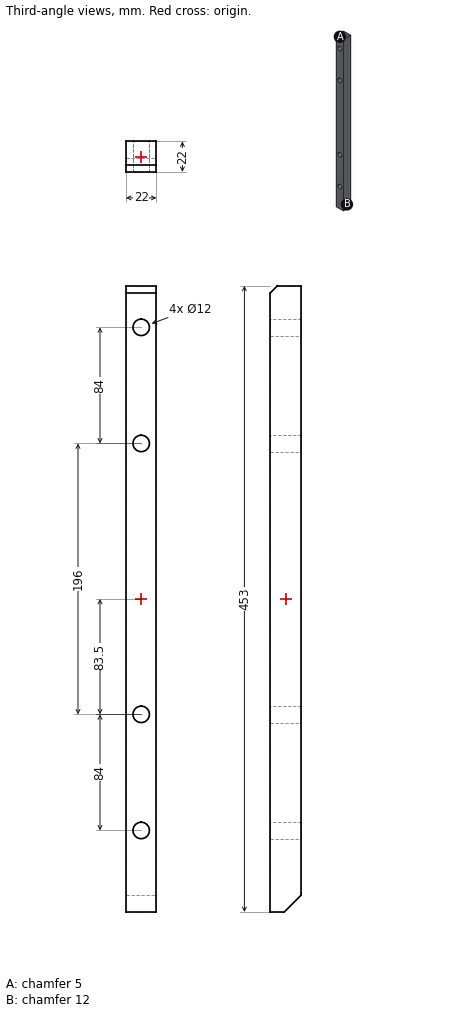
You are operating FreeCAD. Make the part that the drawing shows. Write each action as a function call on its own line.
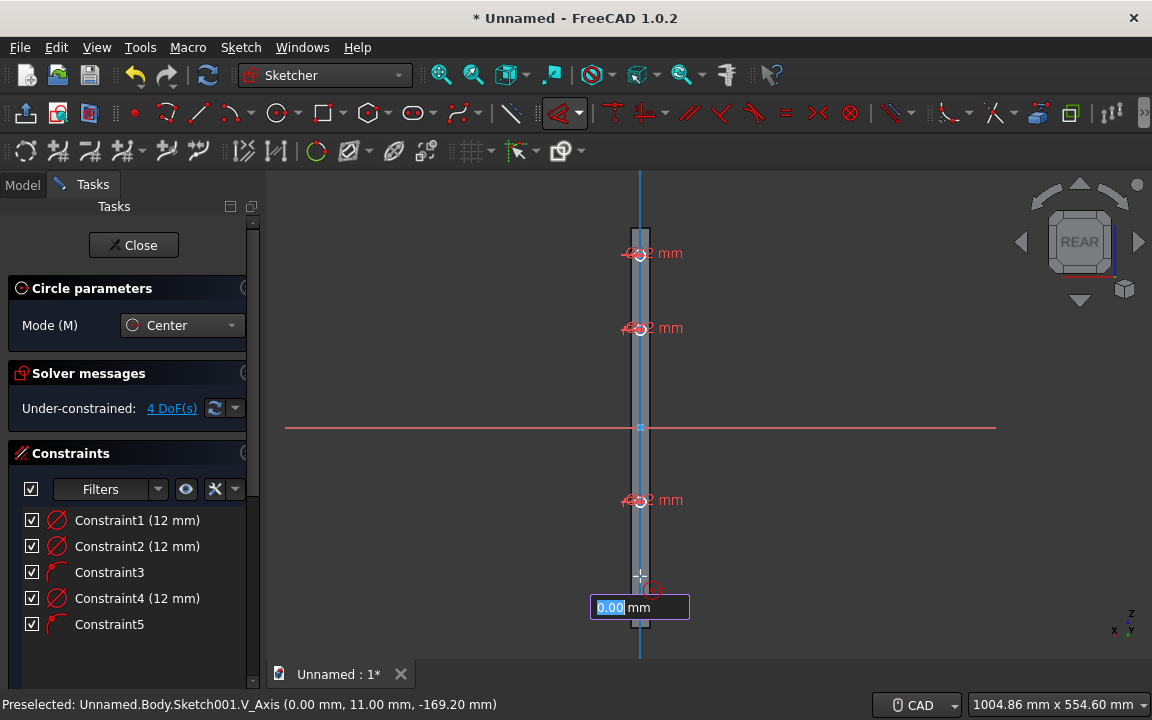
scroll(645, 574, up, 6)
move(646, 571)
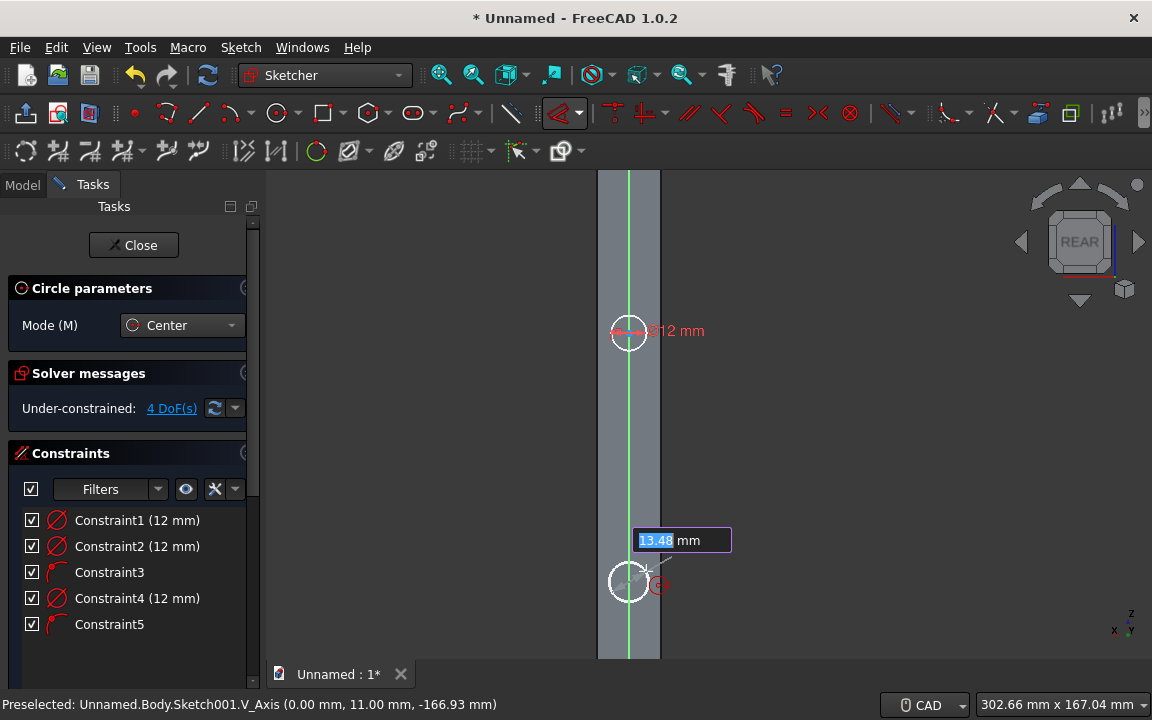
text(12)
key(Return)
key(Escape)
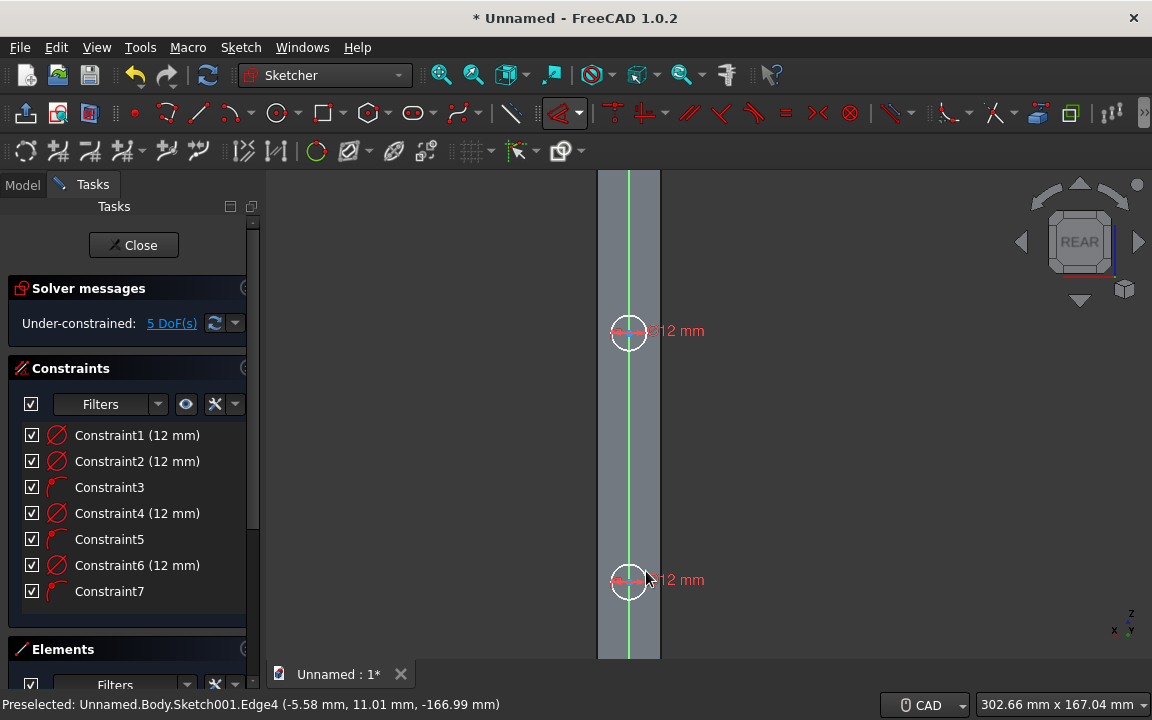
scroll(645, 574, down, 6)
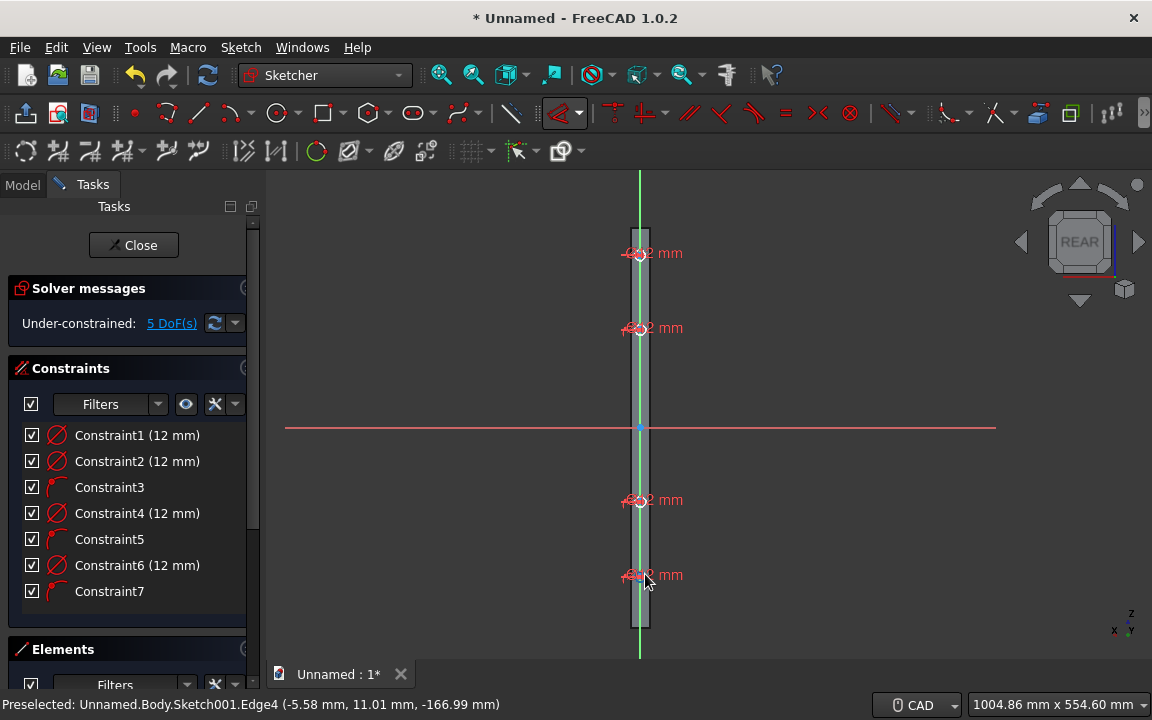
click(640, 255)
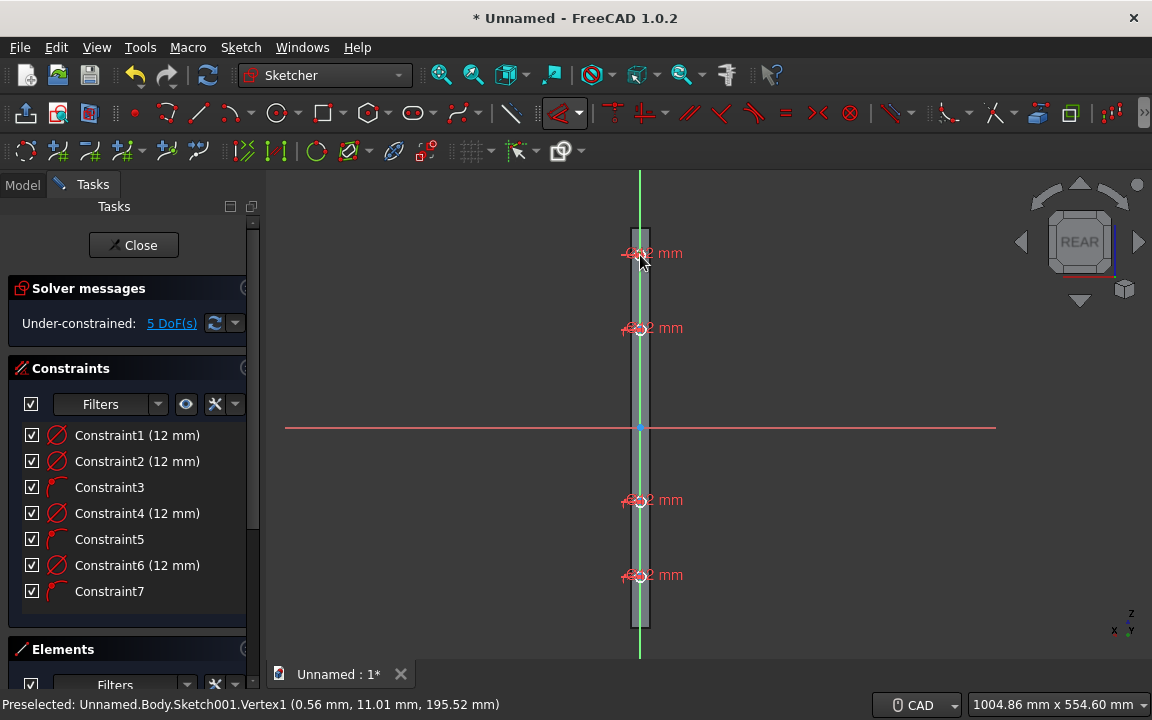
click(640, 538)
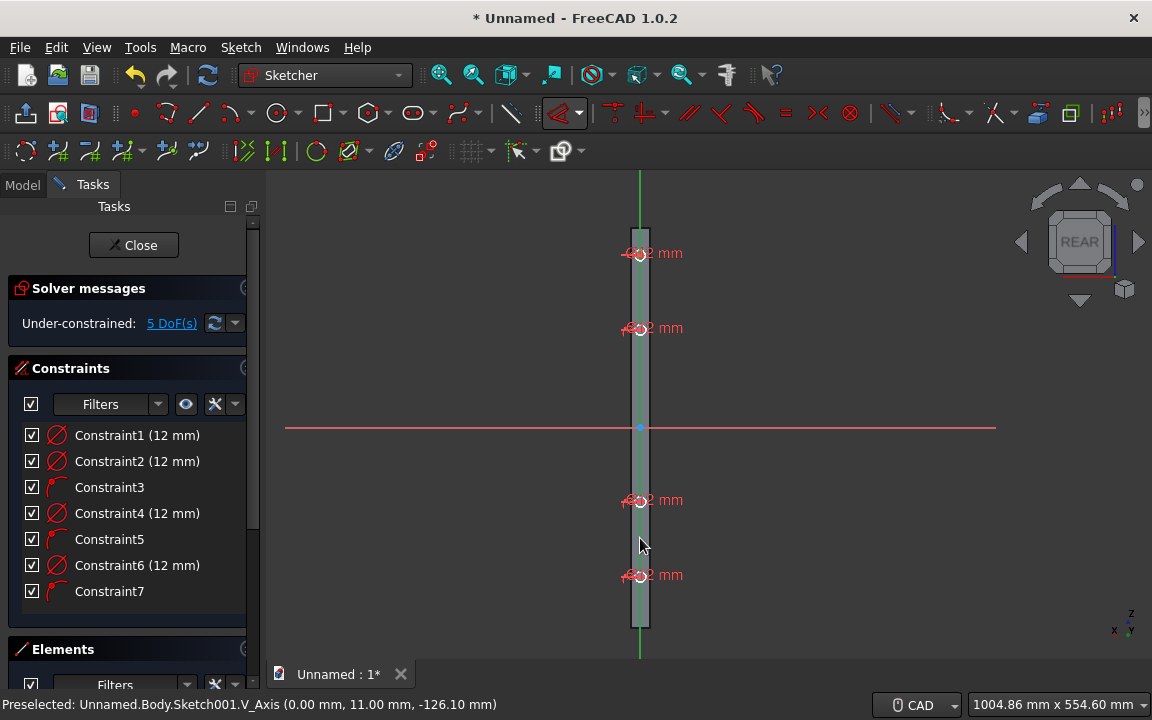
key(c)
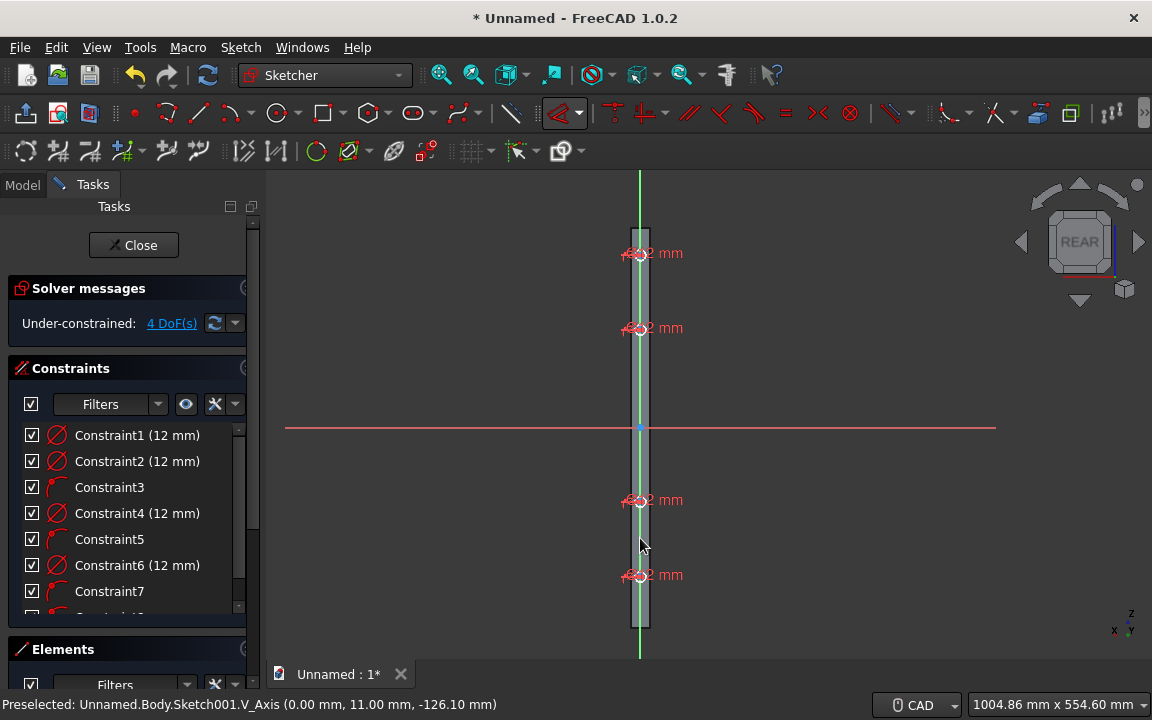
key(d)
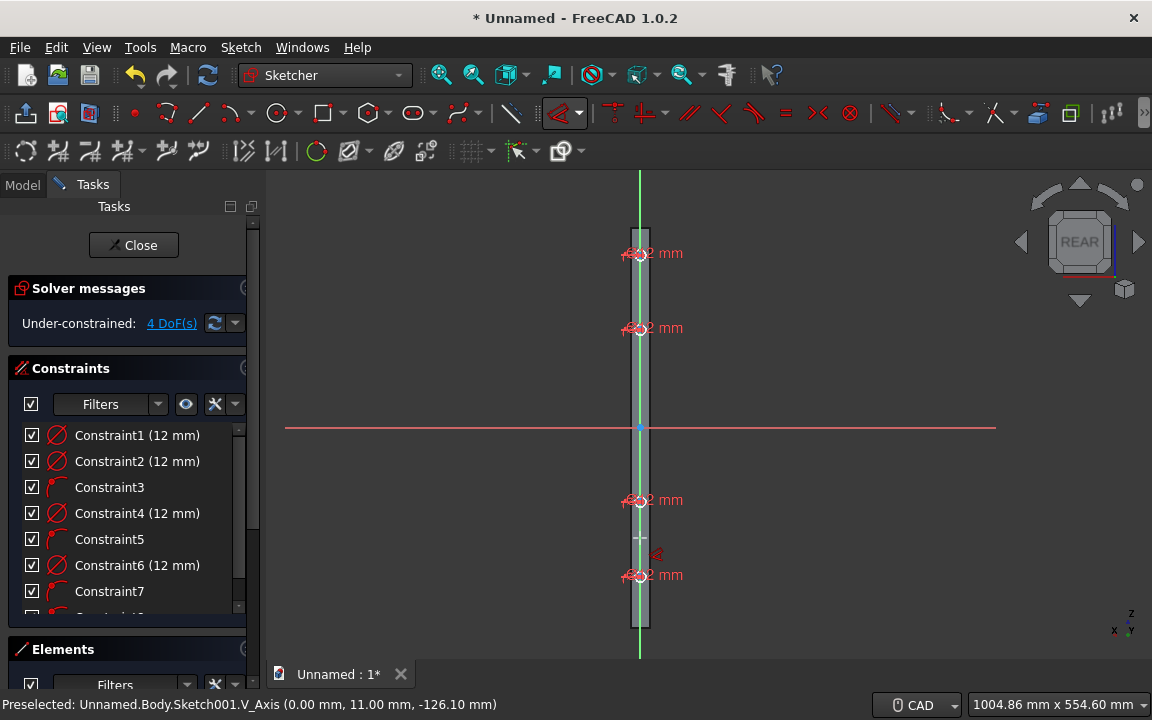
click(640, 255)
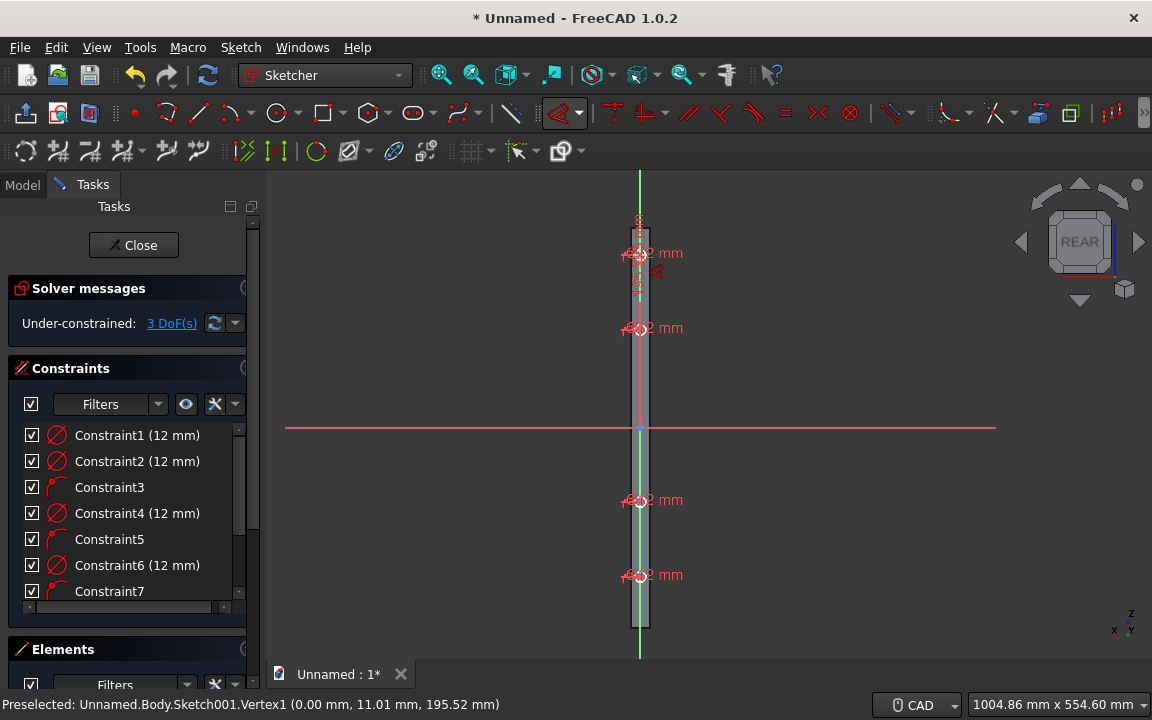
click(640, 330)
click(674, 293)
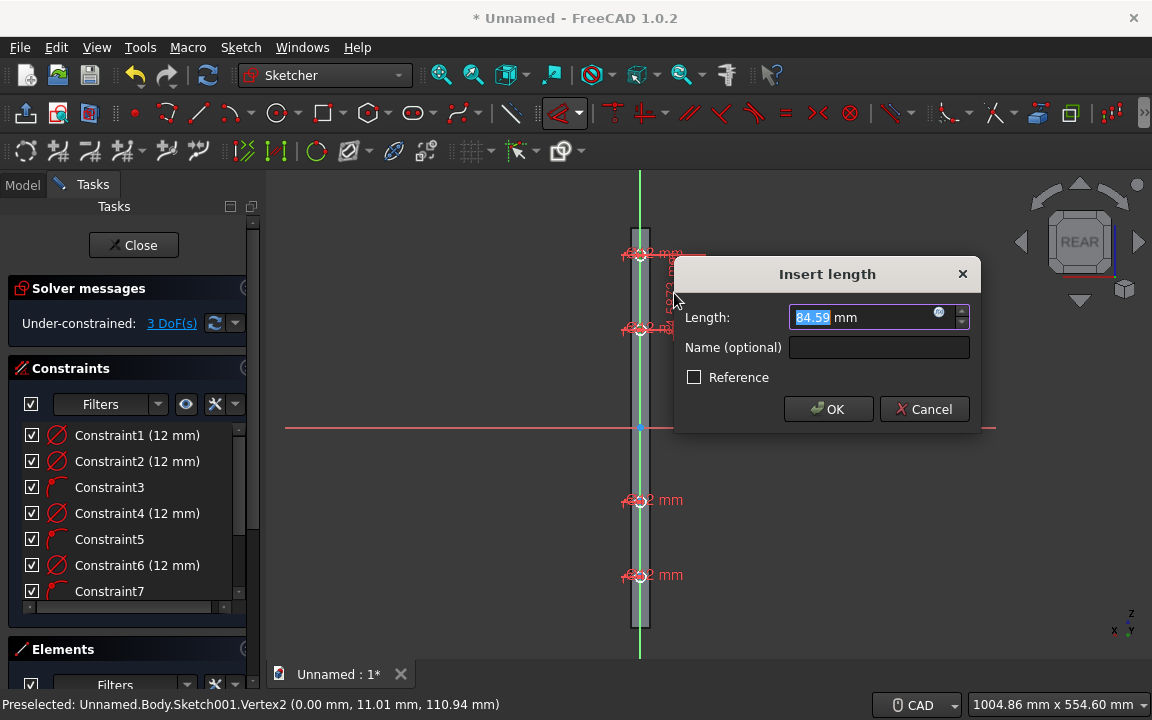
text(84)
key(Return)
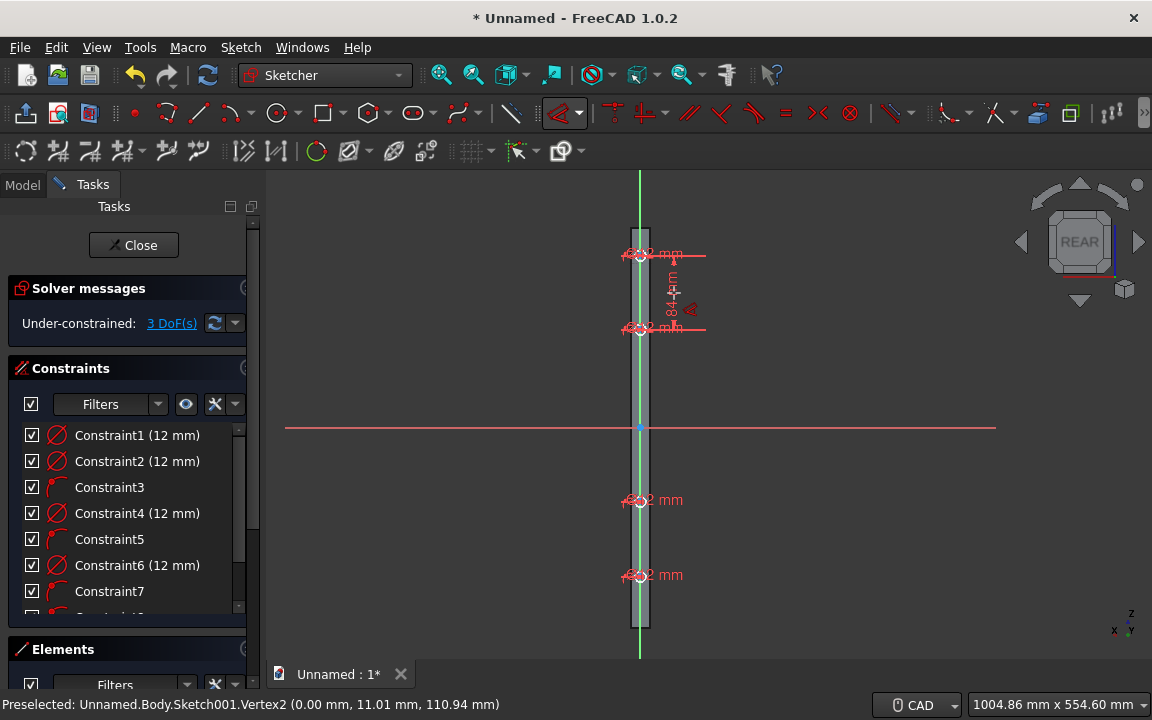
click(640, 502)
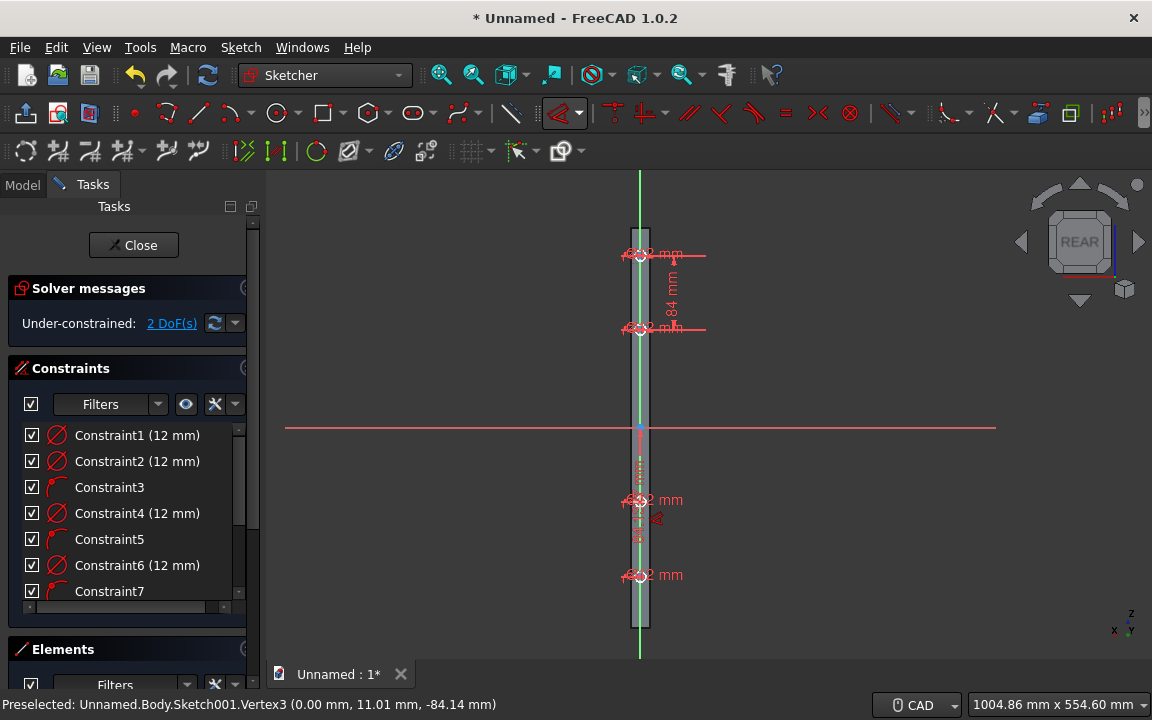
click(640, 577)
click(674, 540)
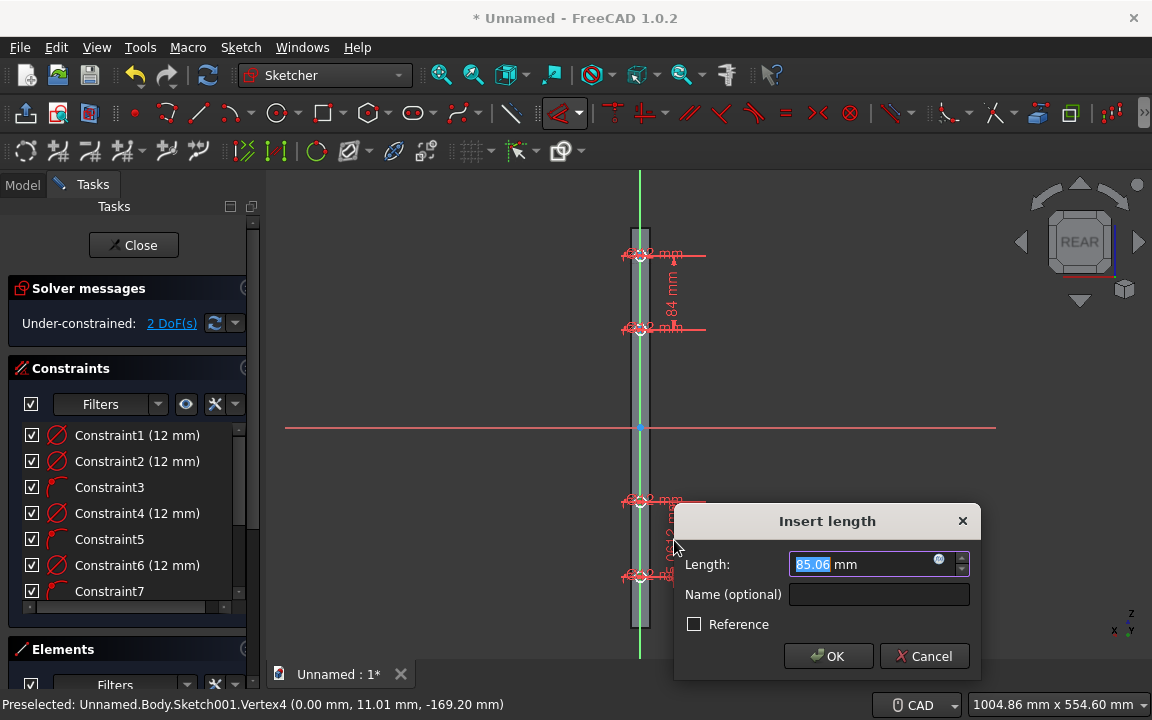
text(84)
key(Return)